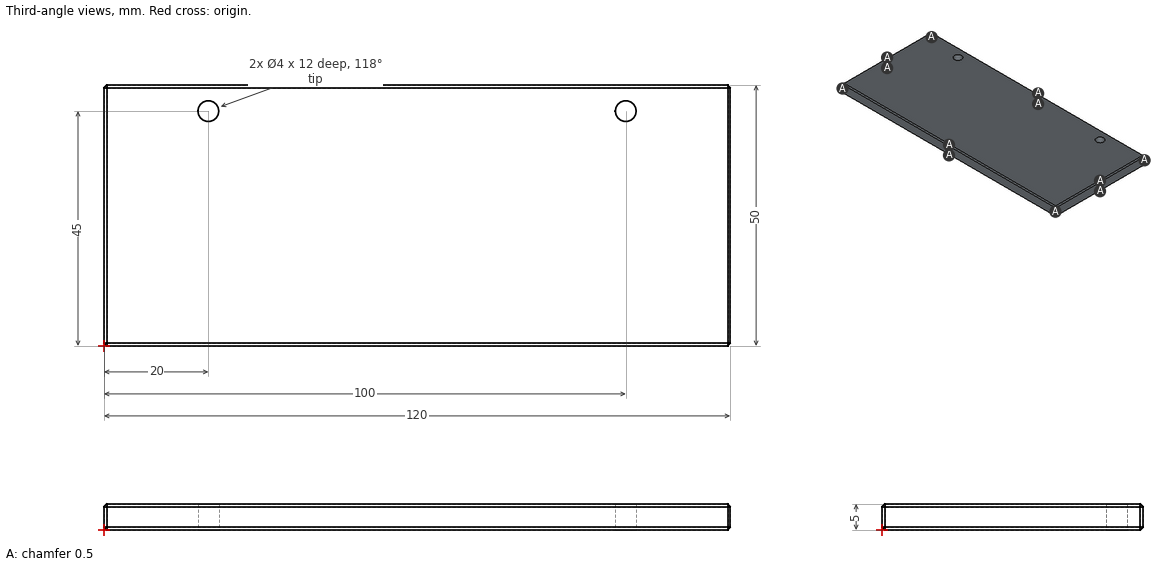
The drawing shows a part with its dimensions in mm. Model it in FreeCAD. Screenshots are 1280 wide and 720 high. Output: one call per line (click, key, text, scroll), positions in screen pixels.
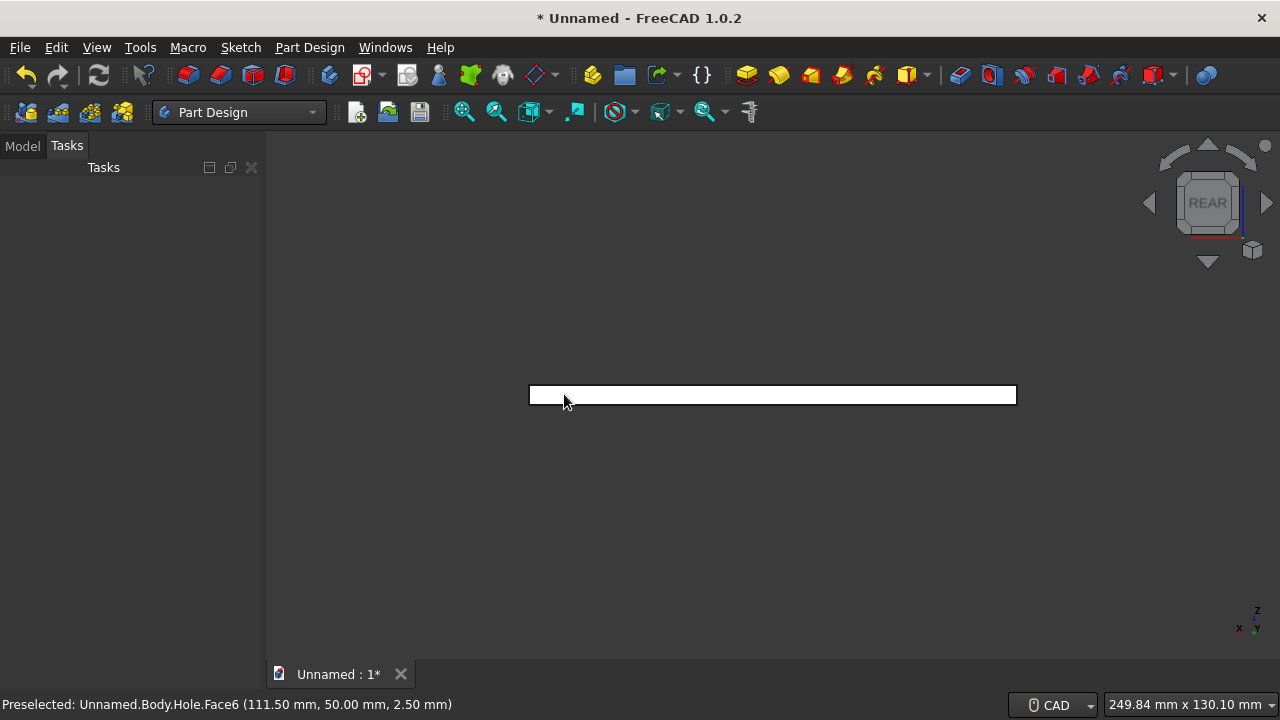
click(222, 76)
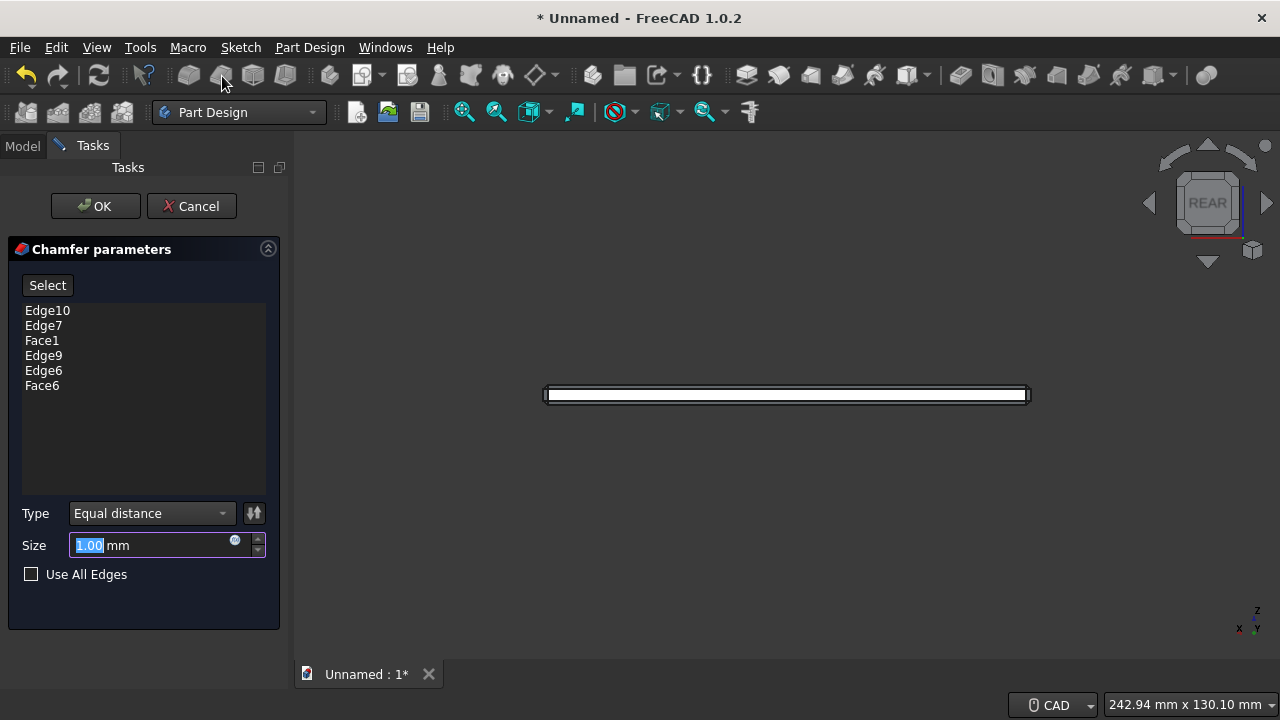
text(0.5)
key(Tab)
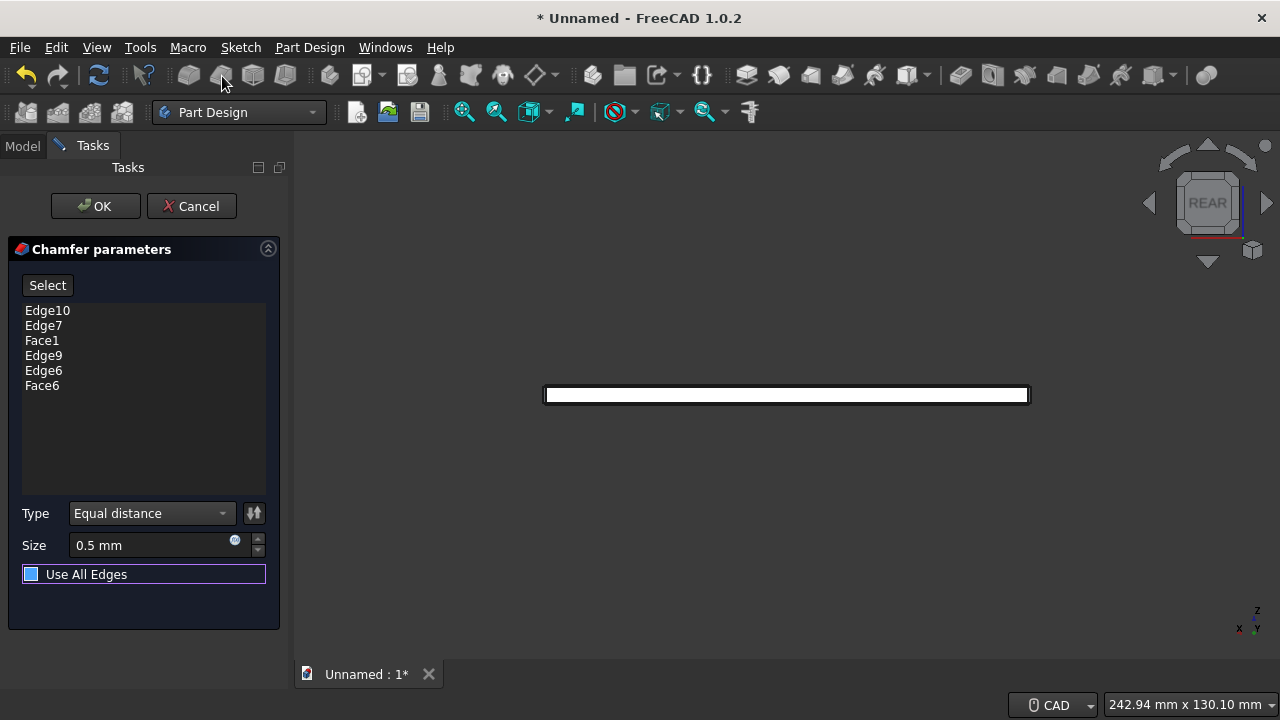
click(96, 206)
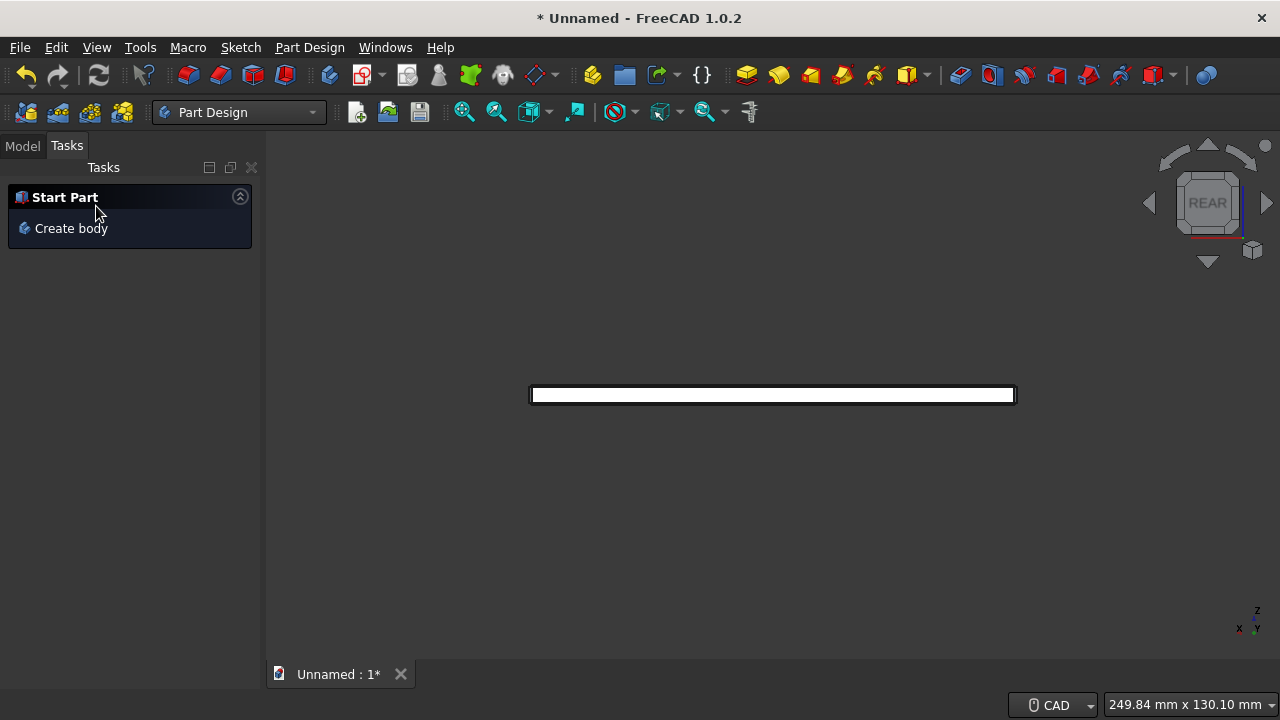
key(0)